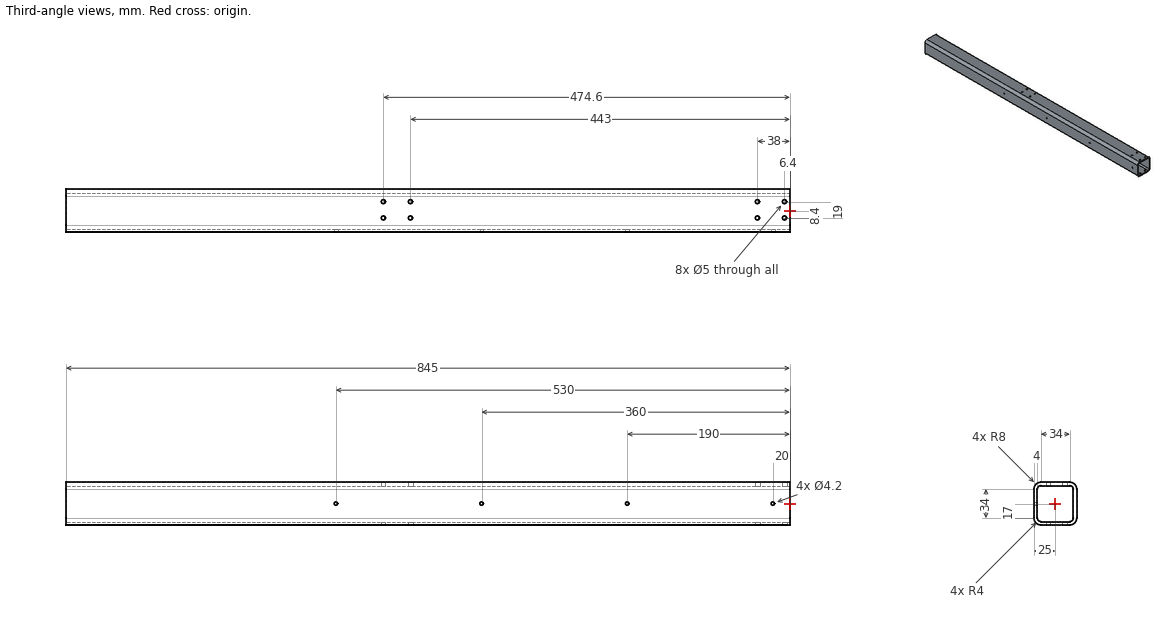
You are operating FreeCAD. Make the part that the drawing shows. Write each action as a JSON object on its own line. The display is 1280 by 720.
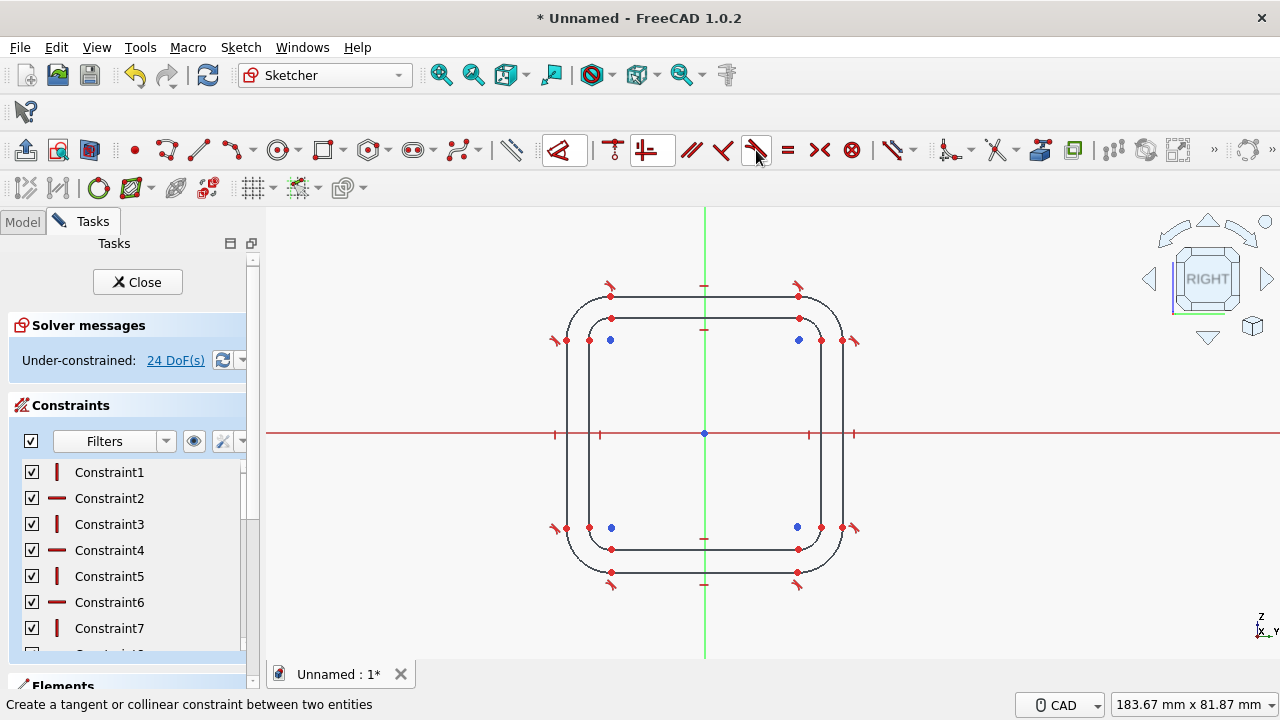
{"action": "left_click", "coordinate": [589, 397]}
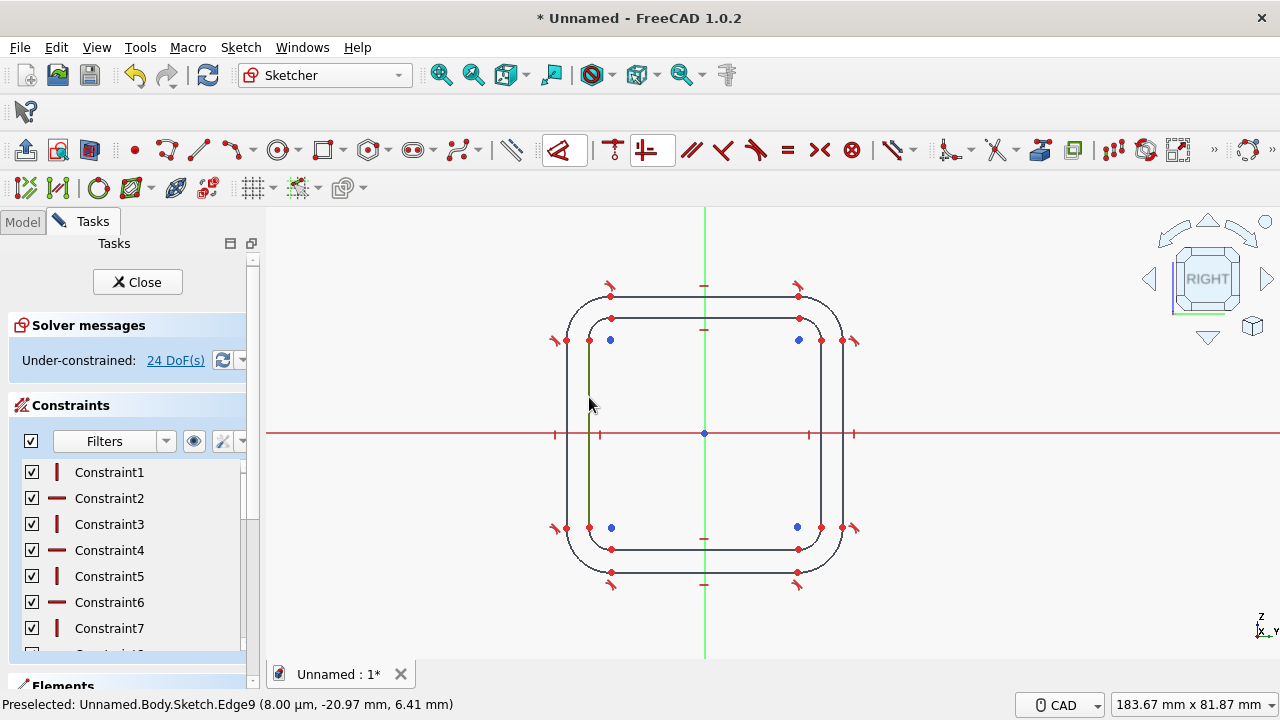
{"action": "scroll", "coordinate": [592, 538], "scroll_direction": "up", "scroll_amount": 2}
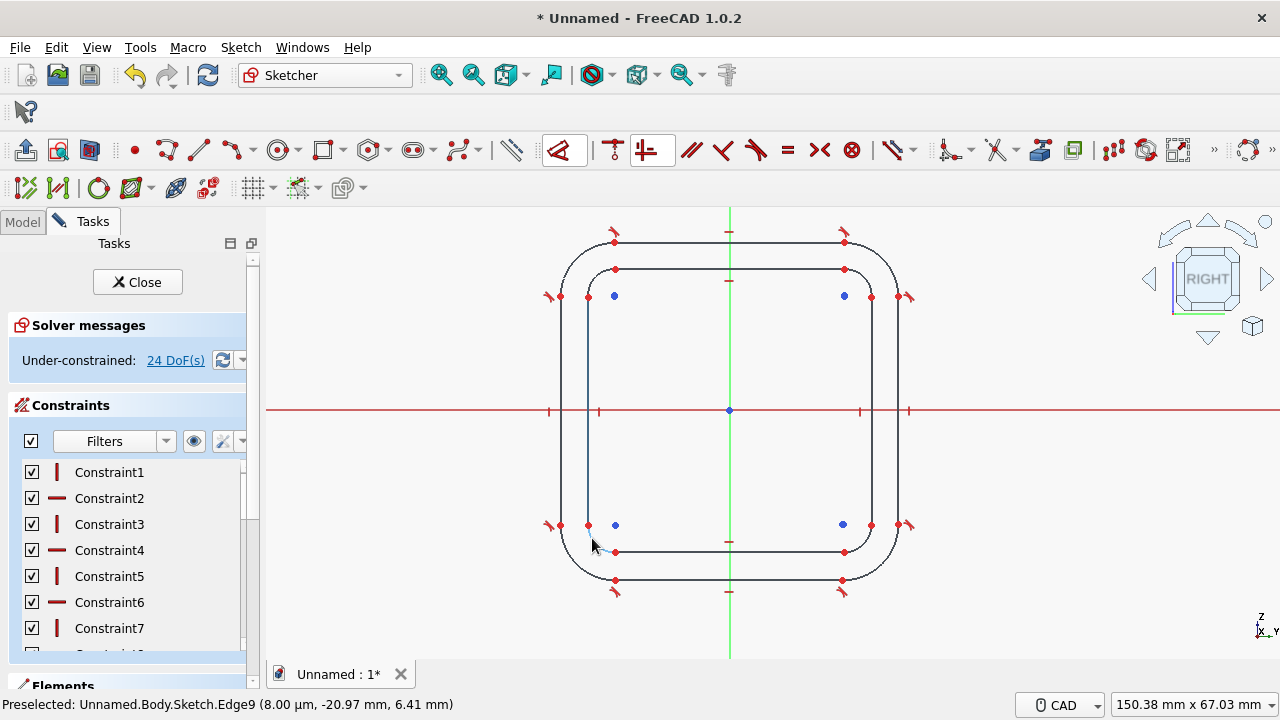
{"action": "left_click", "coordinate": [591, 538]}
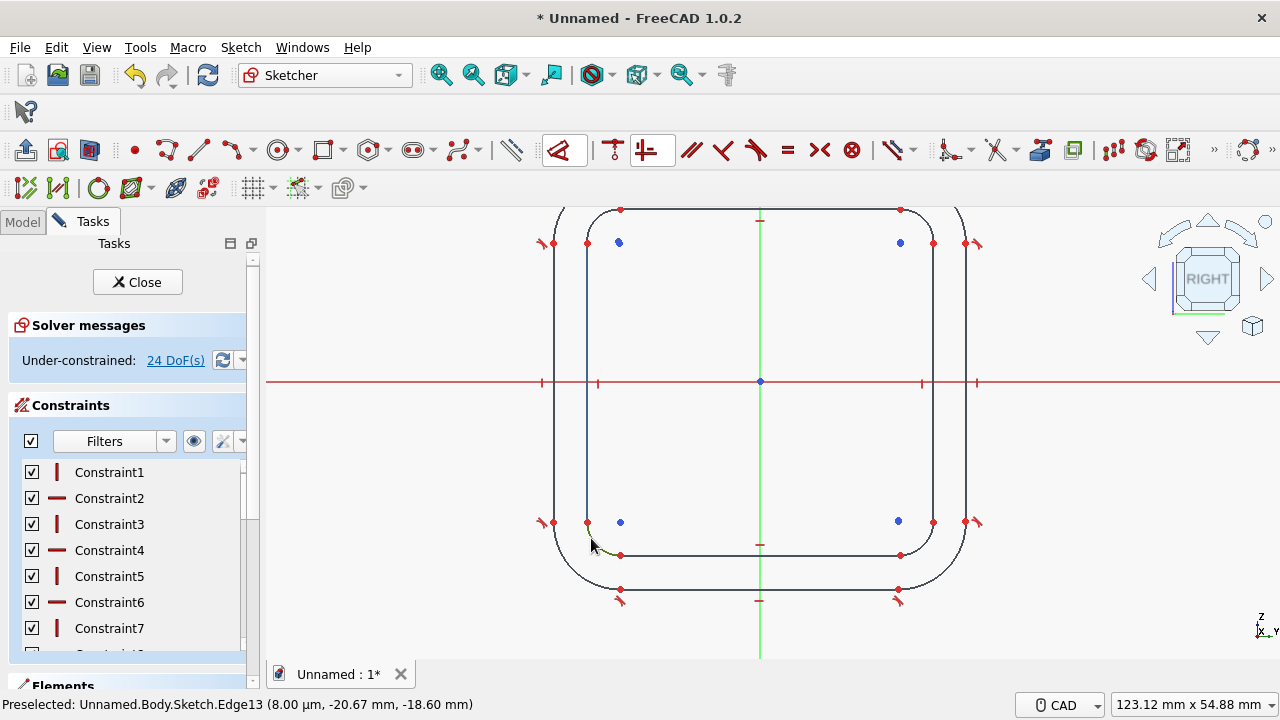
{"action": "left_click", "coordinate": [756, 150]}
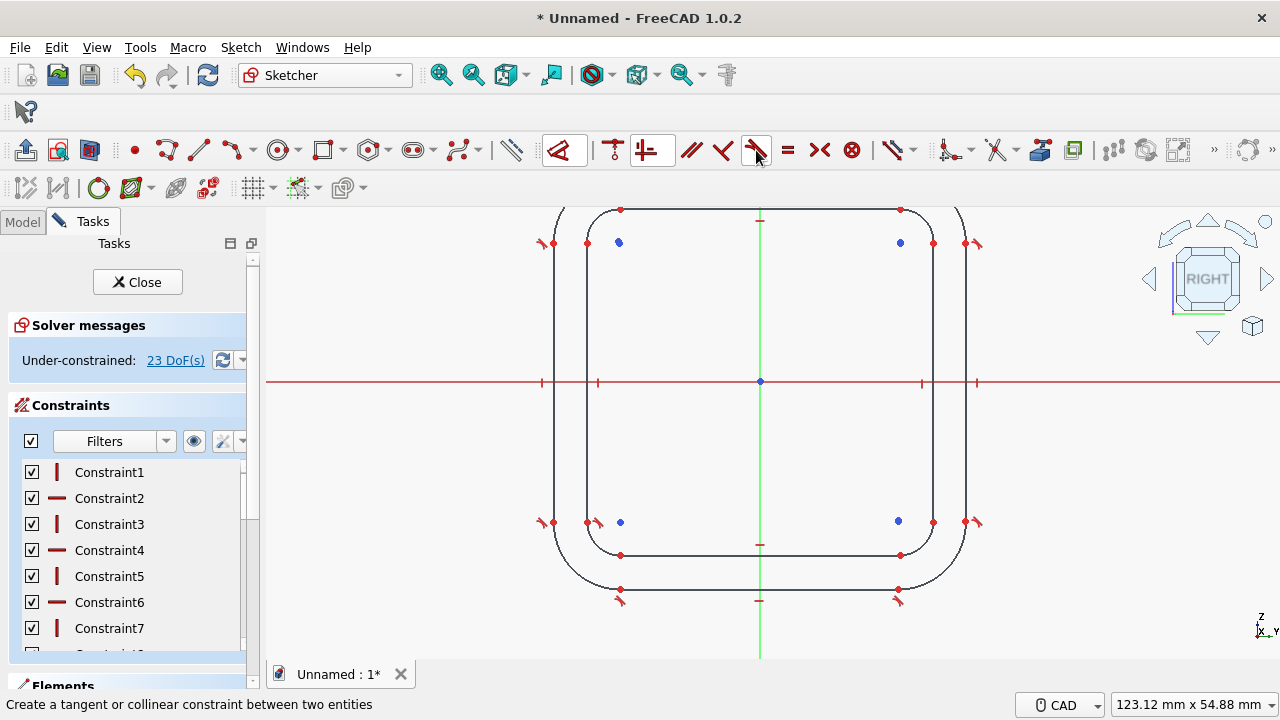
{"action": "left_click", "coordinate": [587, 327]}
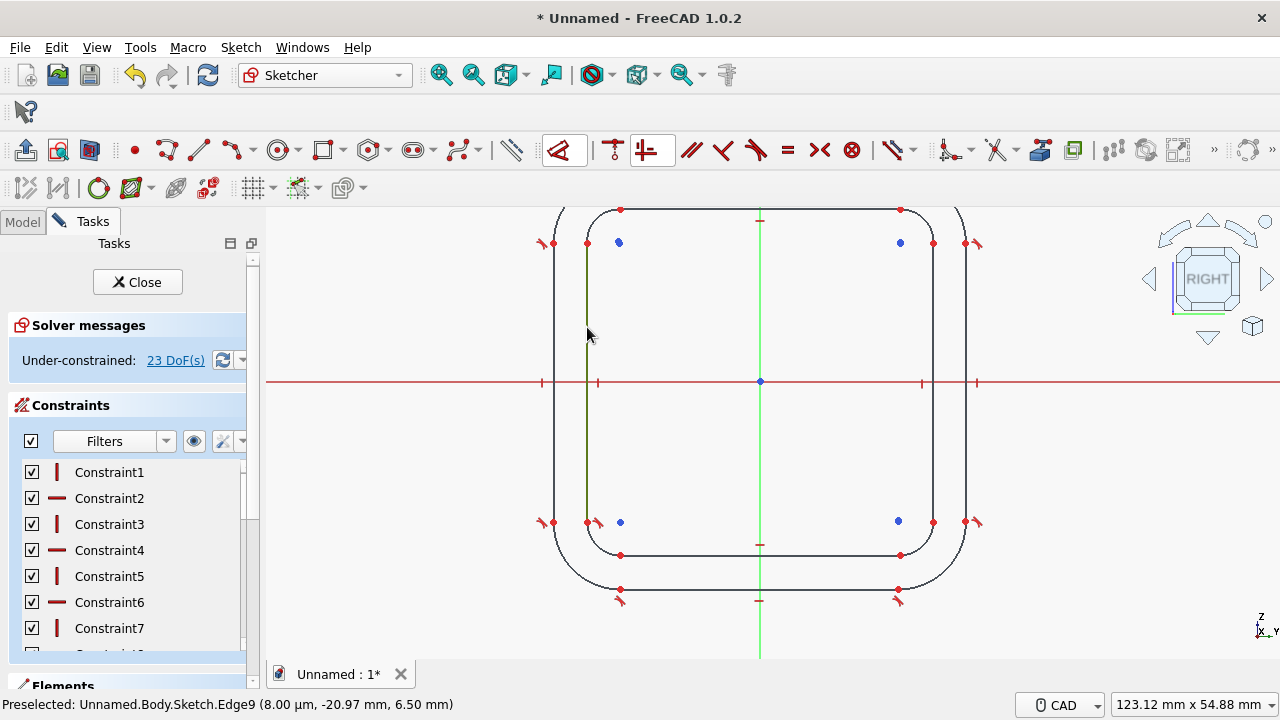
{"action": "scroll", "coordinate": [592, 538], "scroll_direction": "down", "scroll_amount": 2}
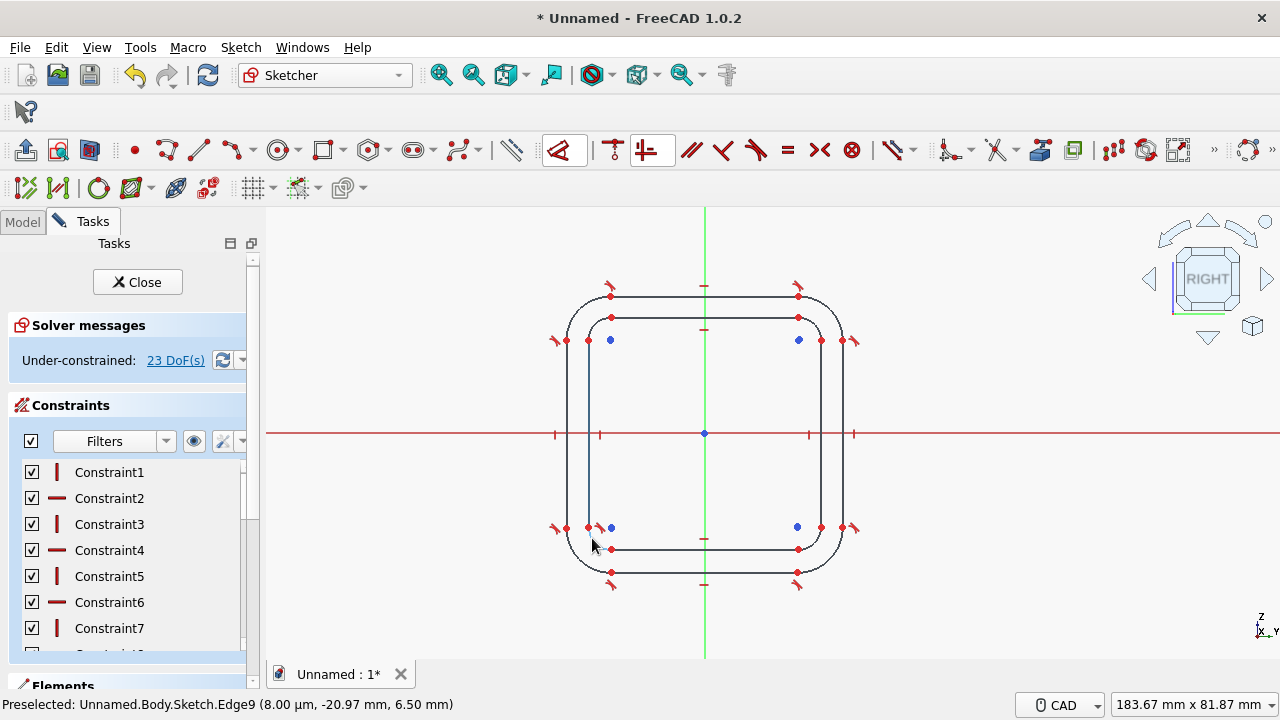
{"action": "scroll", "coordinate": [601, 320], "scroll_direction": "up", "scroll_amount": 2}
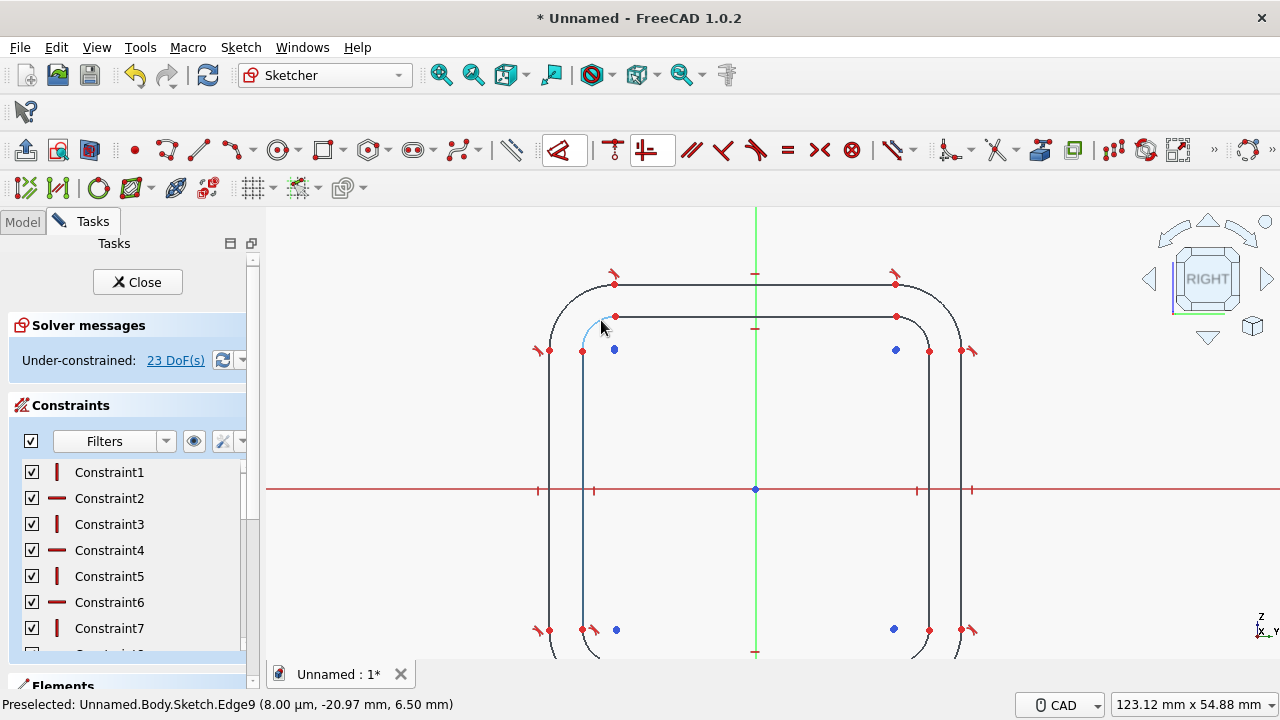
{"action": "left_click", "coordinate": [600, 320]}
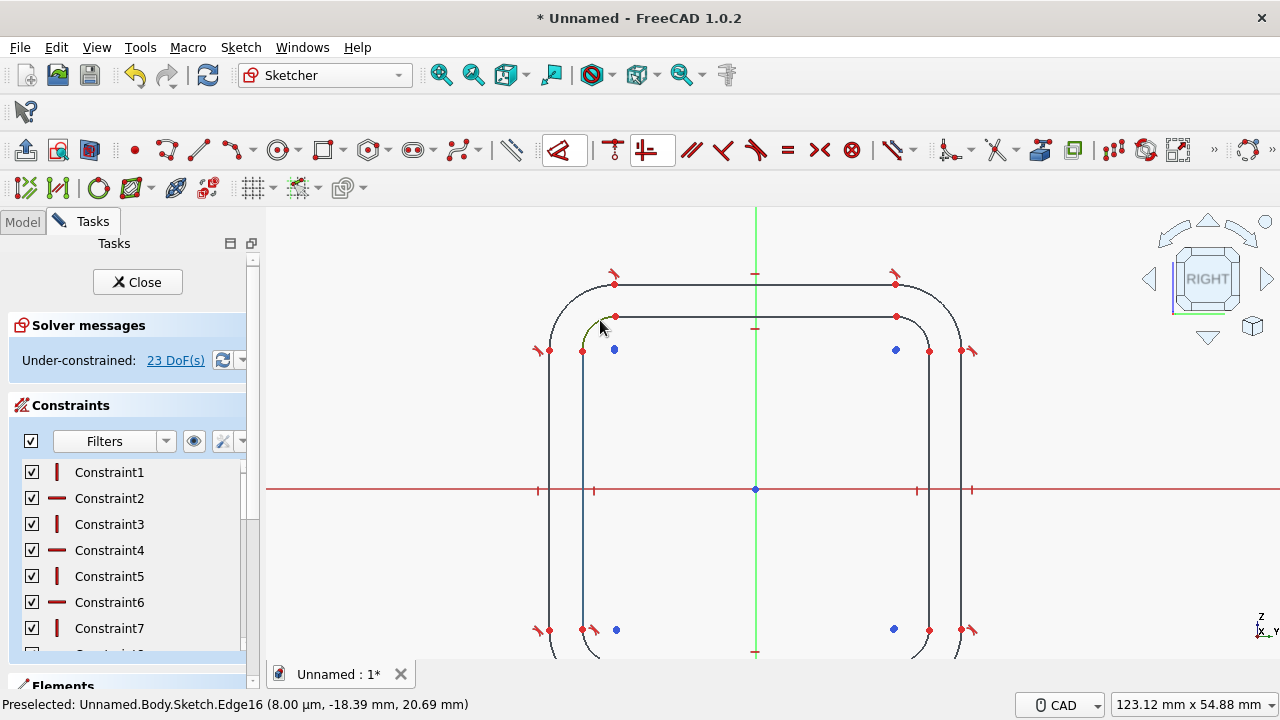
{"action": "left_click", "coordinate": [756, 150]}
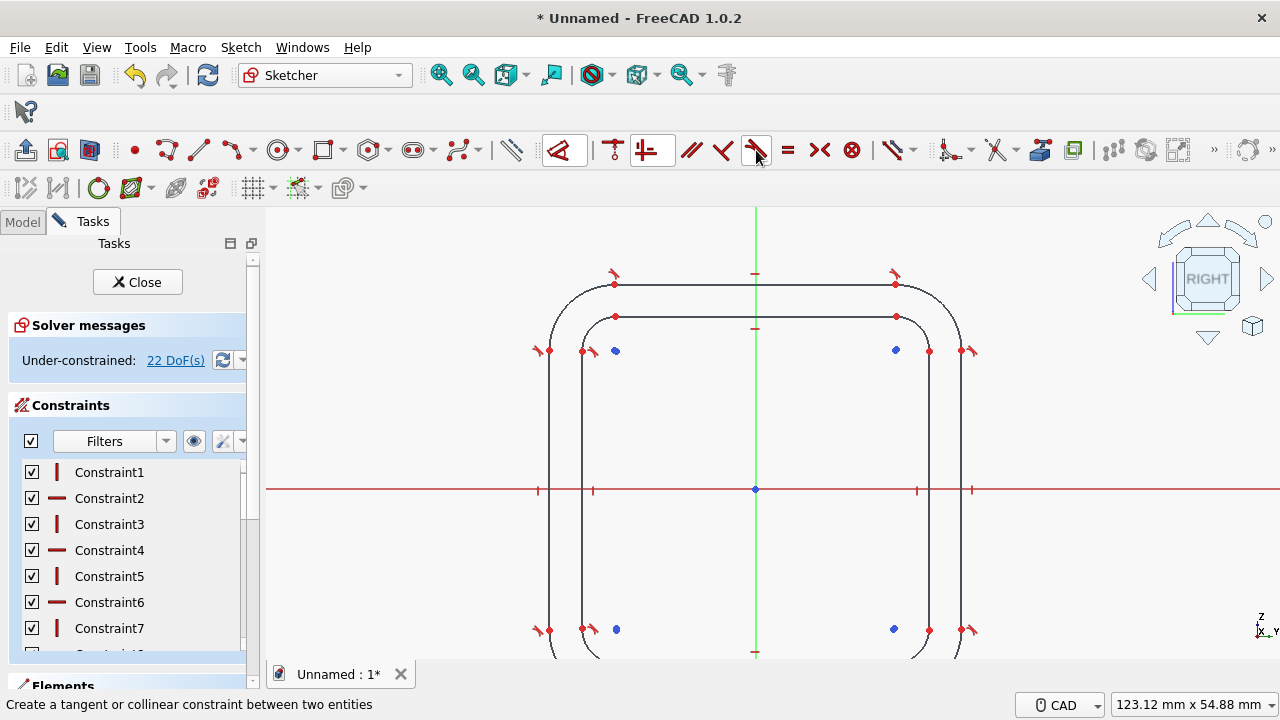
{"action": "scroll", "coordinate": [601, 319], "scroll_direction": "down", "scroll_amount": 2}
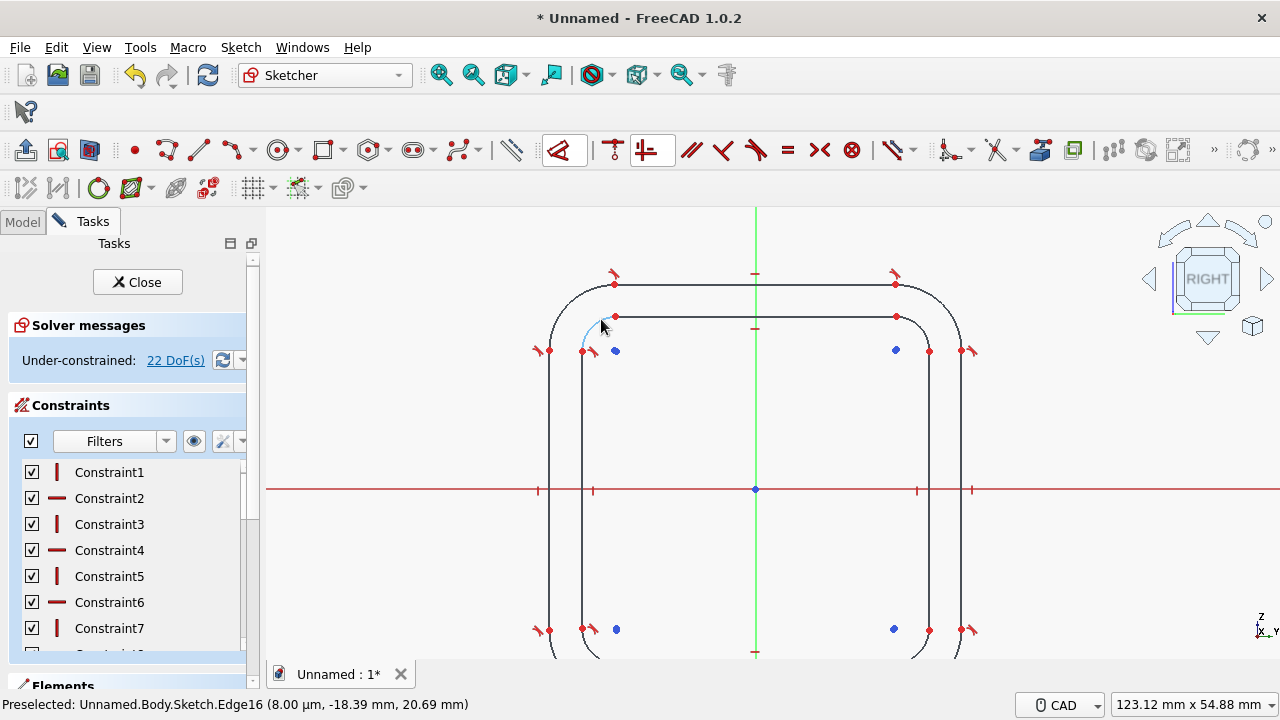
{"action": "left_click", "coordinate": [667, 550]}